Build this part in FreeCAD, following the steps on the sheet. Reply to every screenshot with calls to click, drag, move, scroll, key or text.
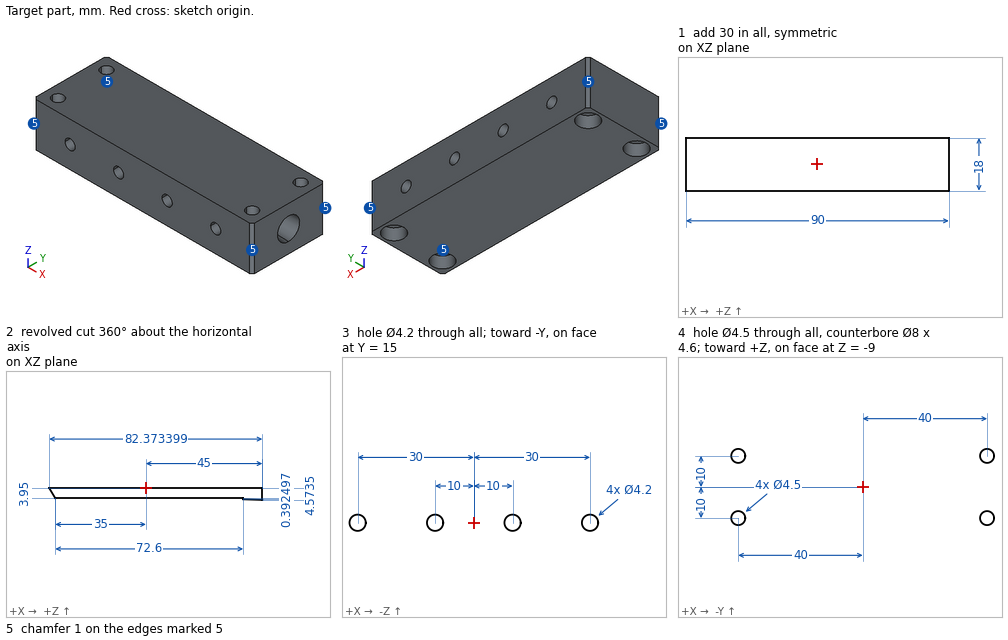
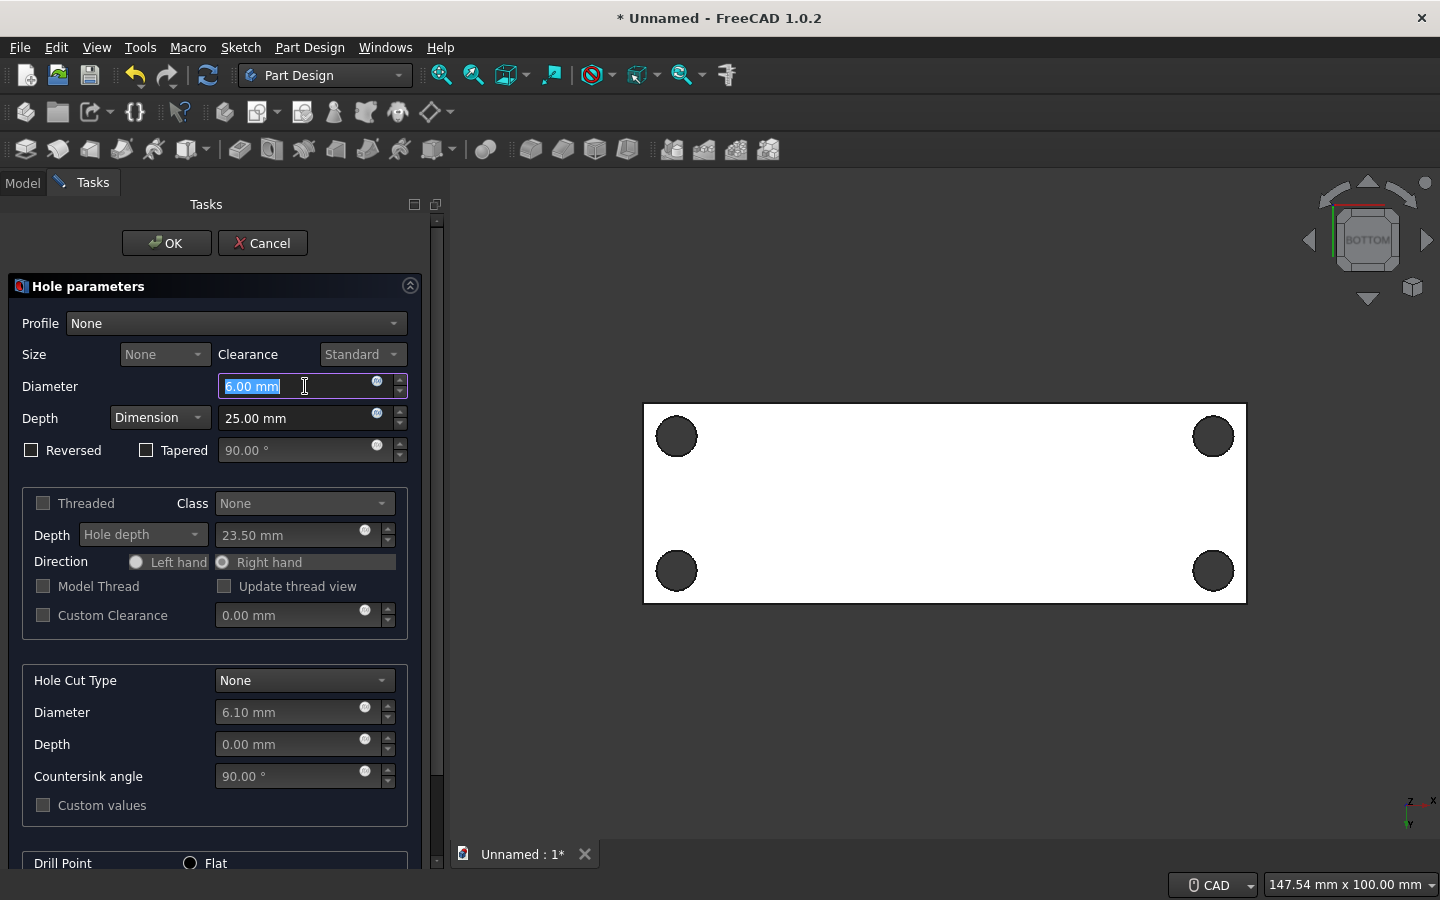
text(4.5)
key(Tab)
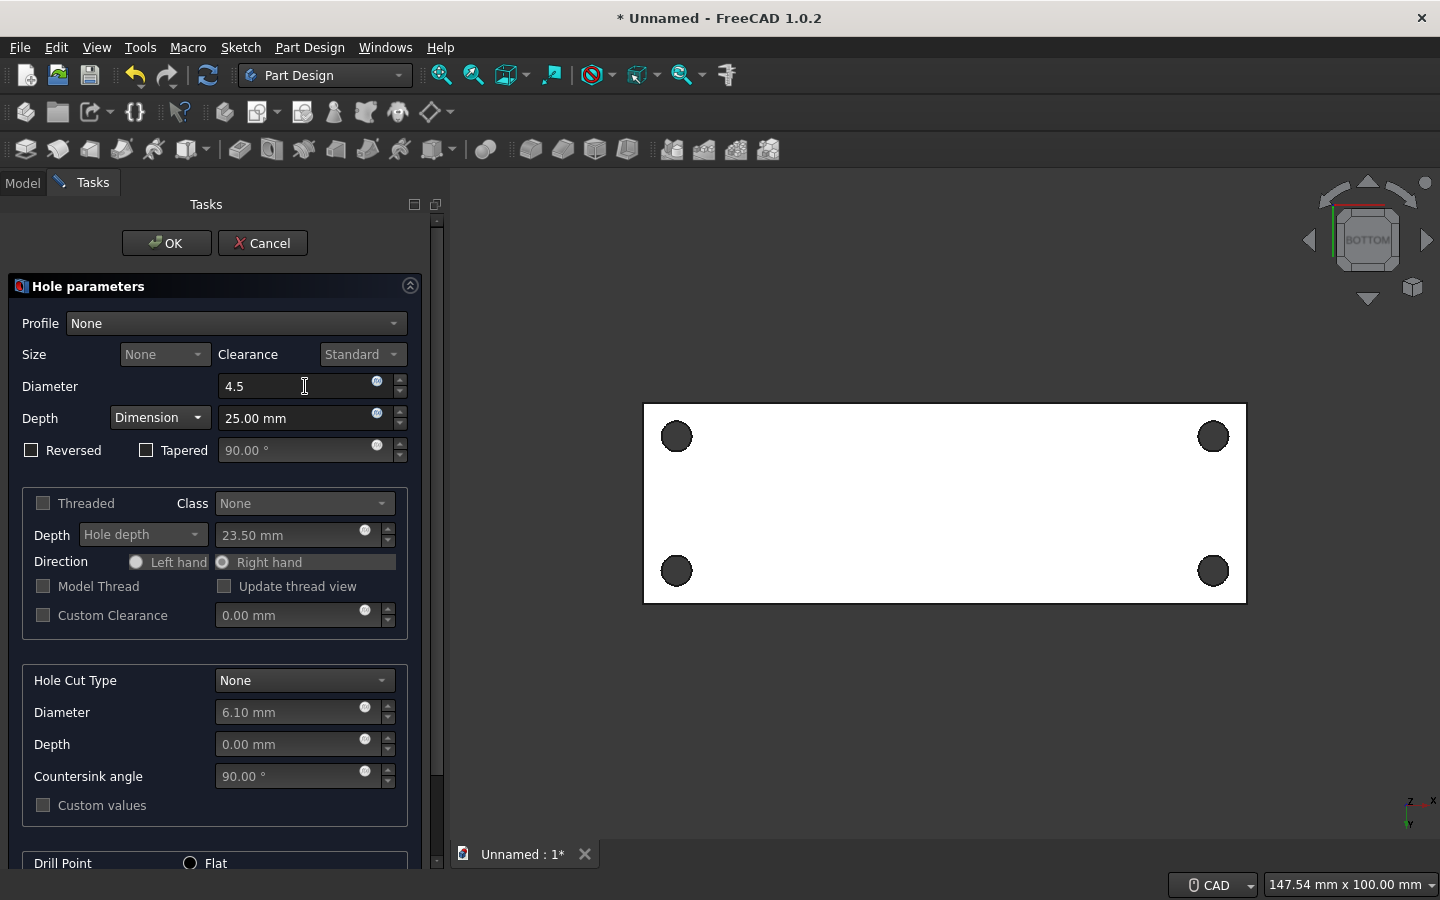
click(161, 418)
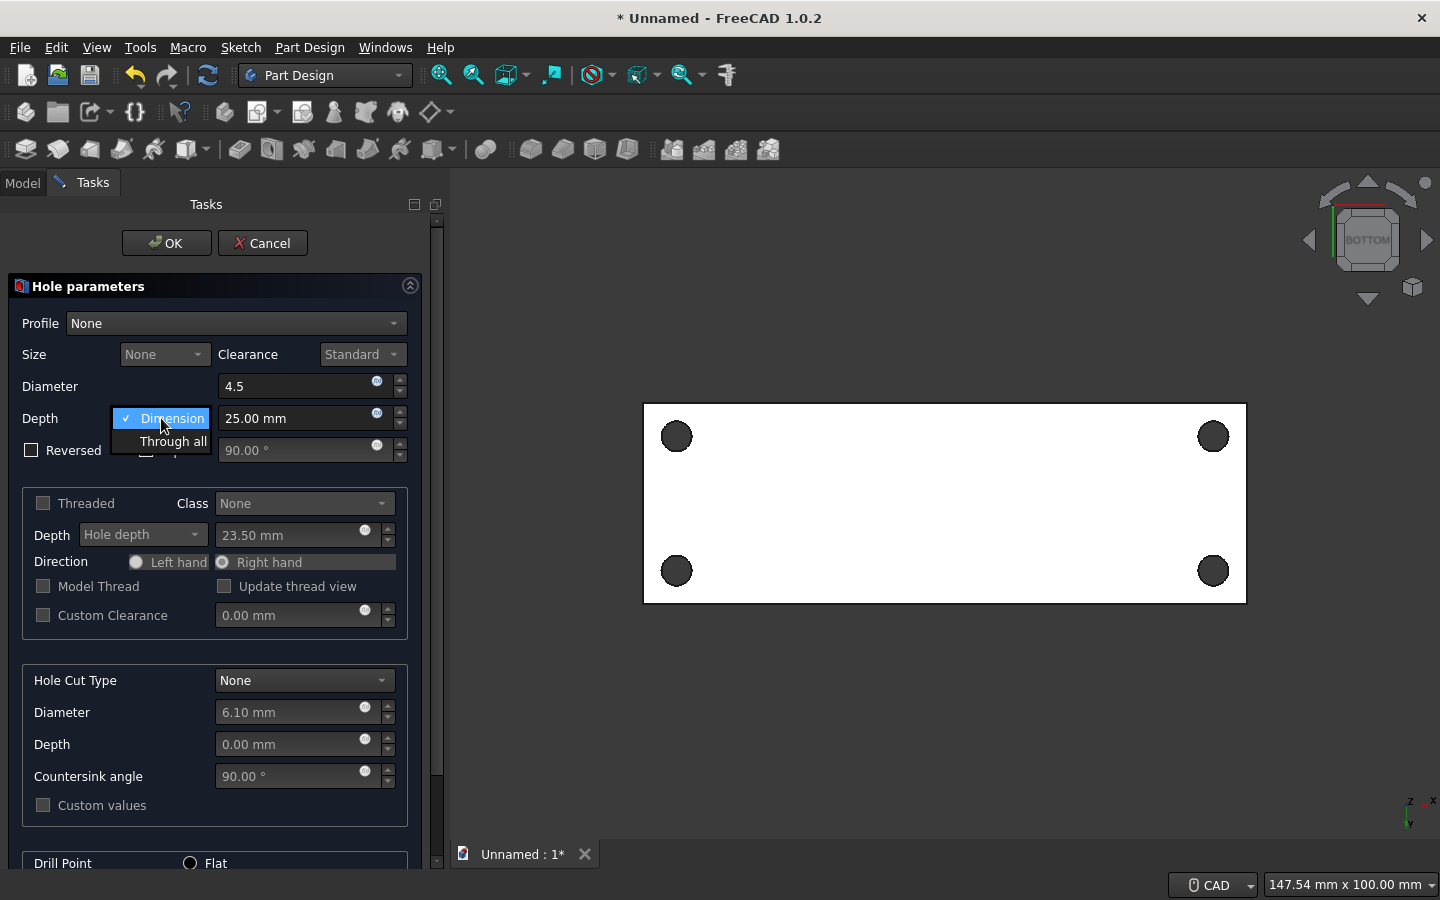
click(160, 442)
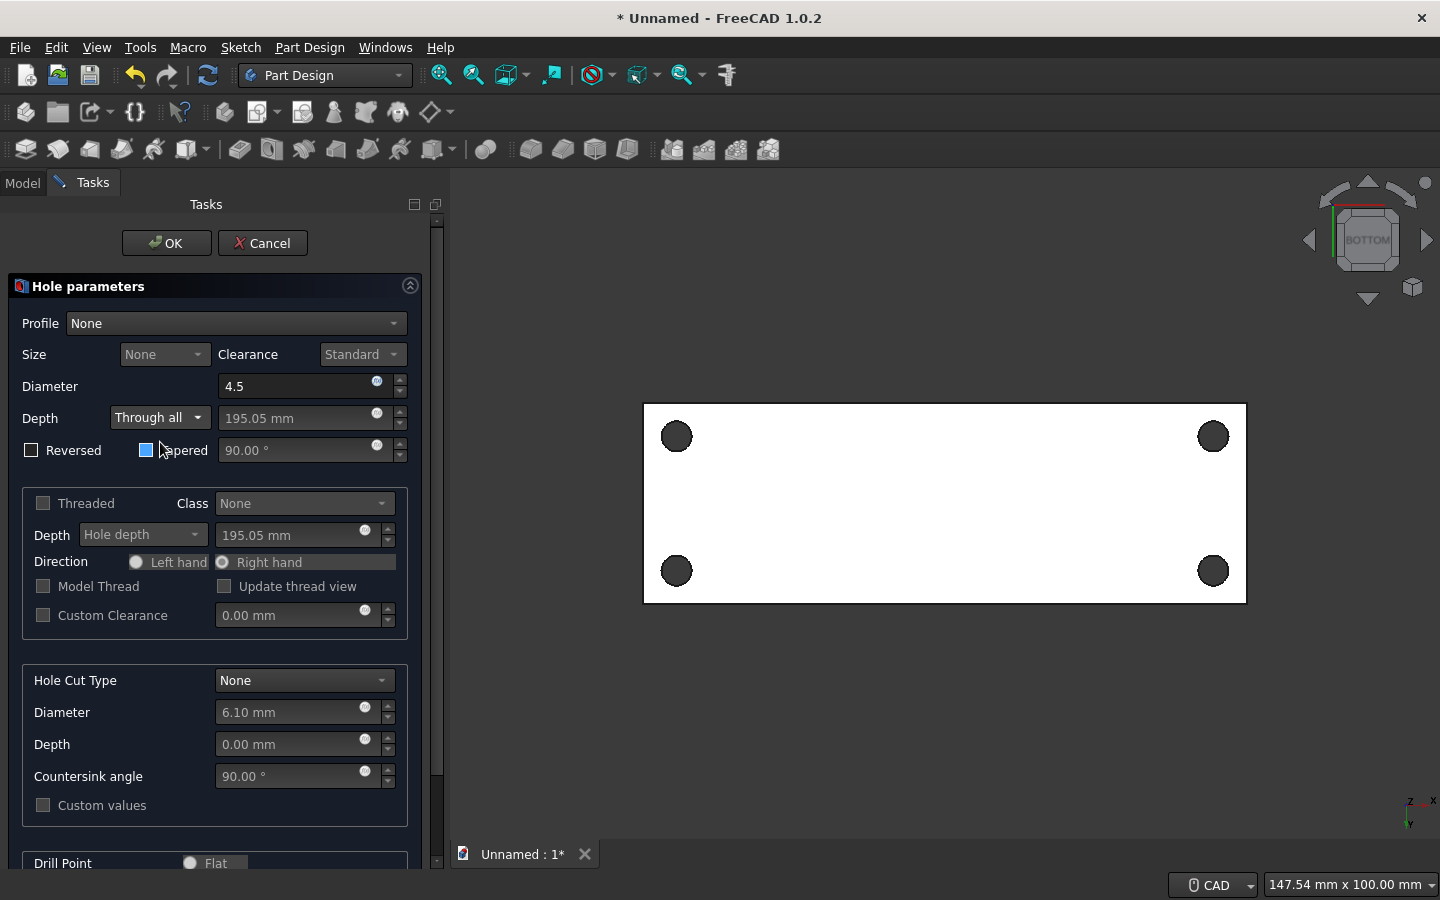
click(306, 680)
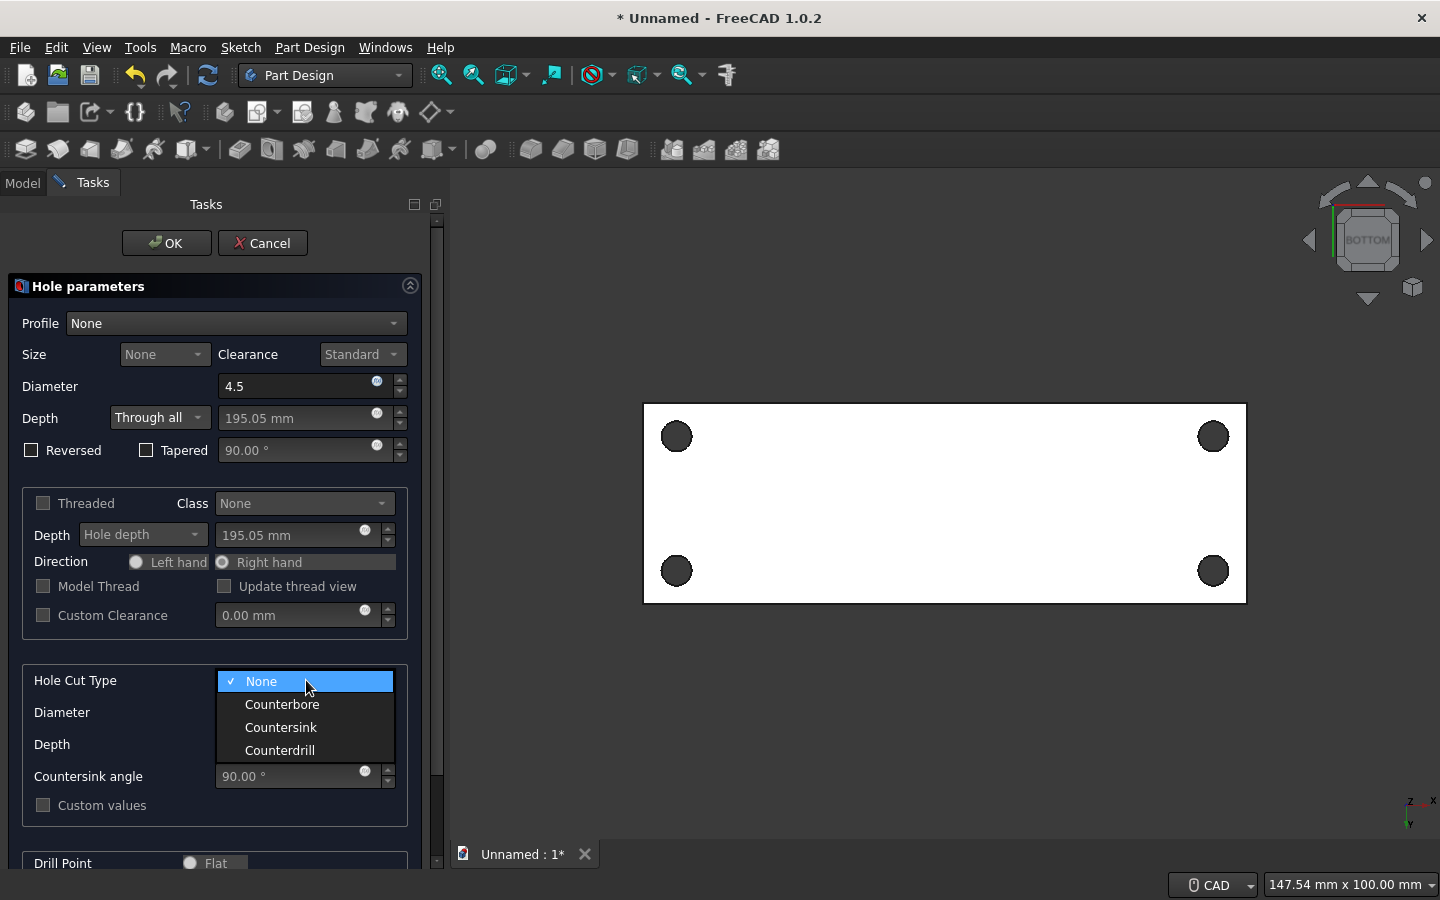
click(304, 704)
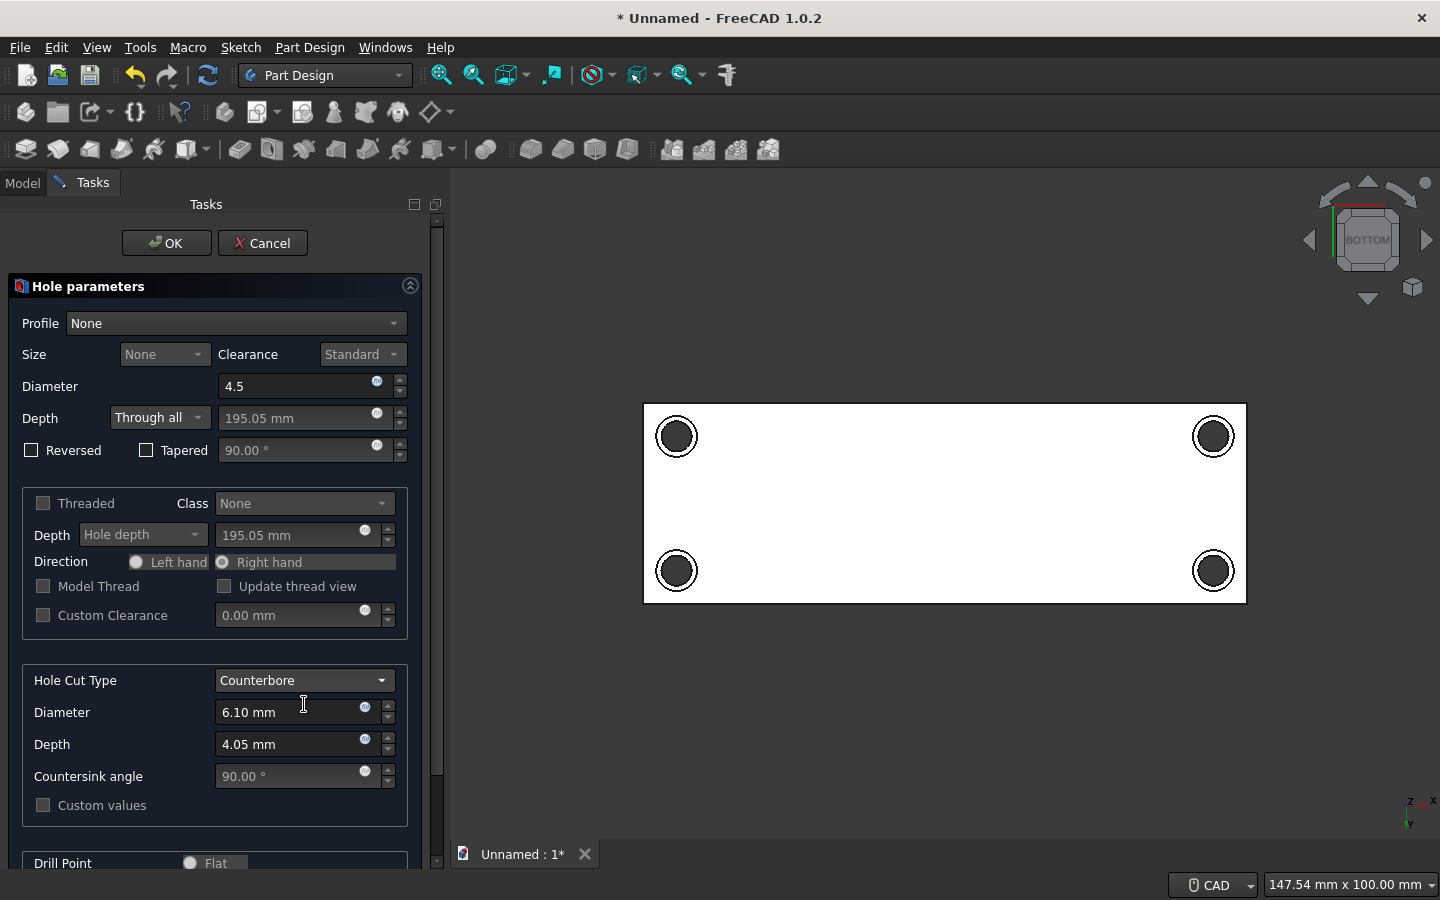
triple_click(298, 712)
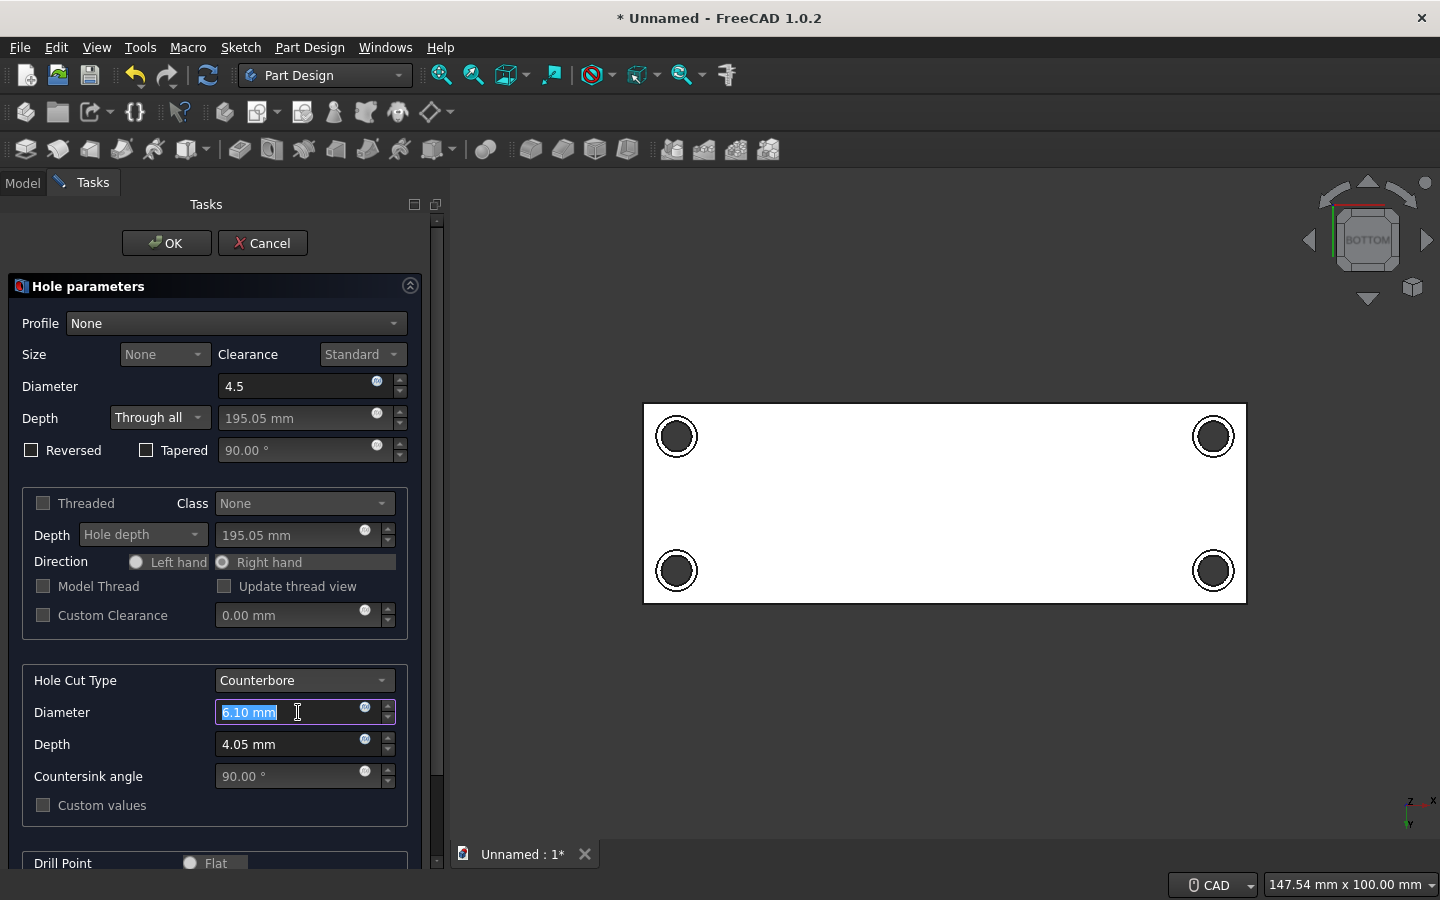
text(8)
key(Tab)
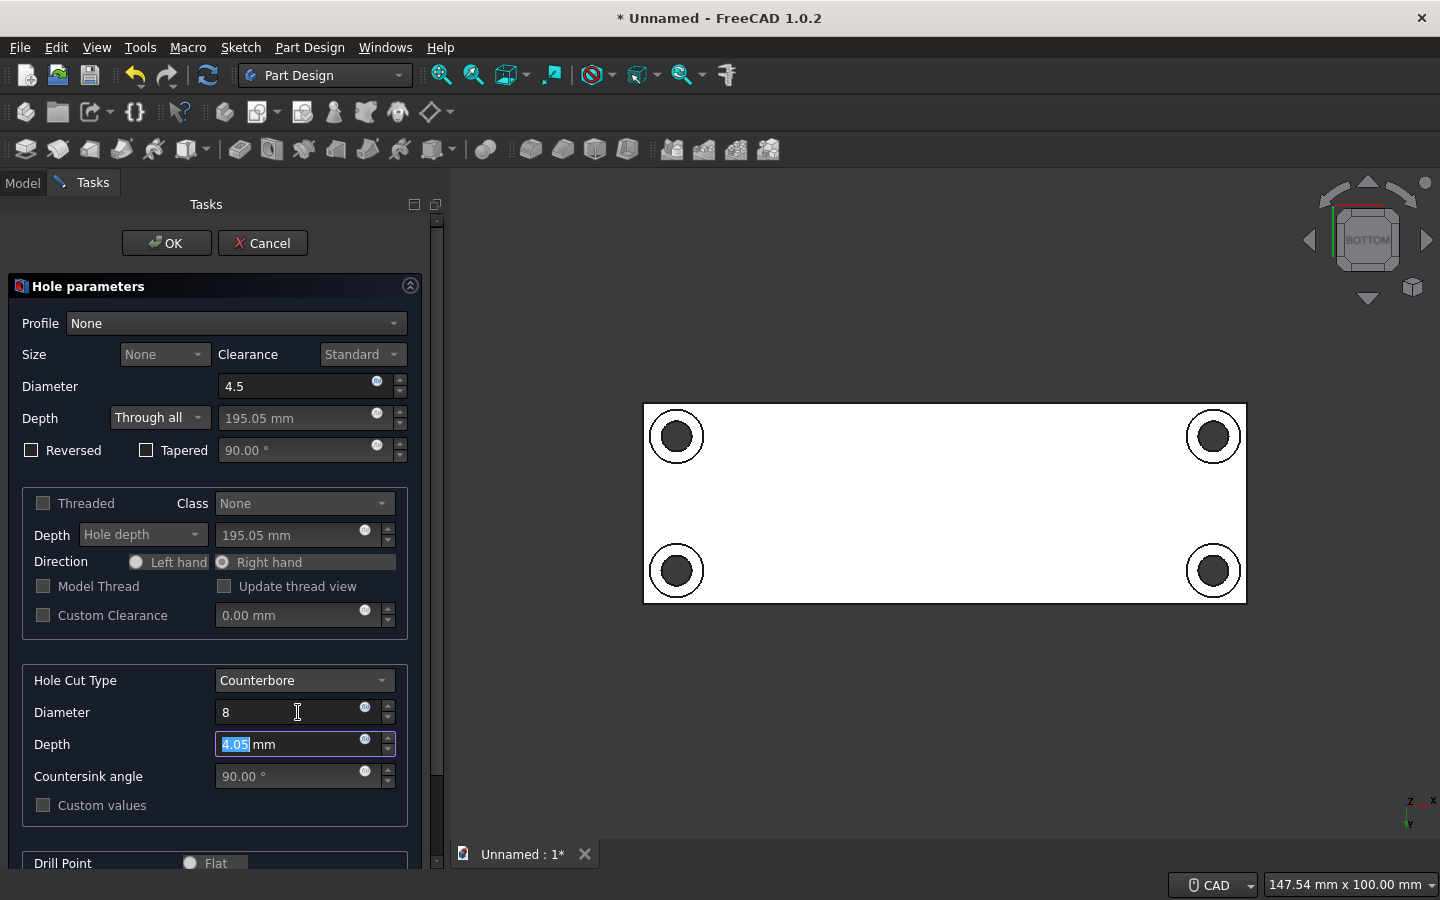
text(4.6)
key(Tab)